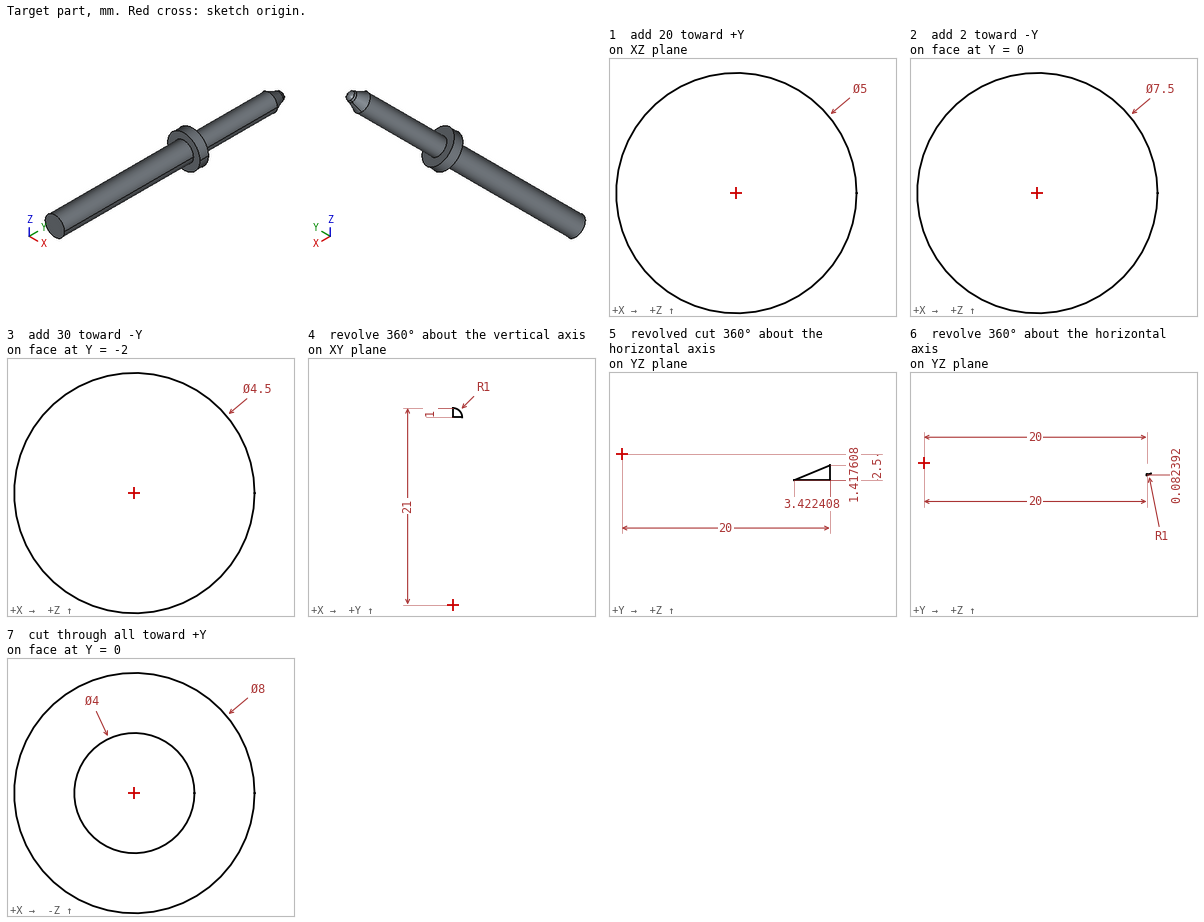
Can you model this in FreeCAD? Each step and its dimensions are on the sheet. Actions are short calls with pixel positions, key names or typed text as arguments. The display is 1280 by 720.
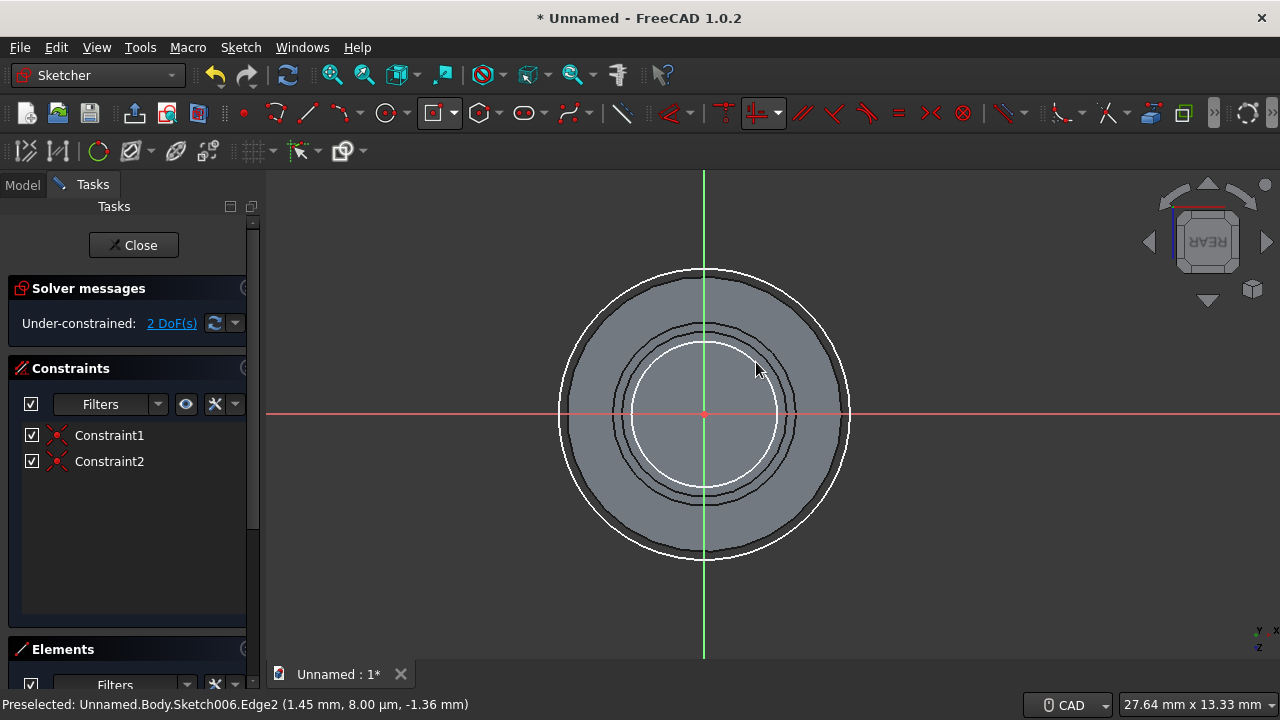
click(670, 114)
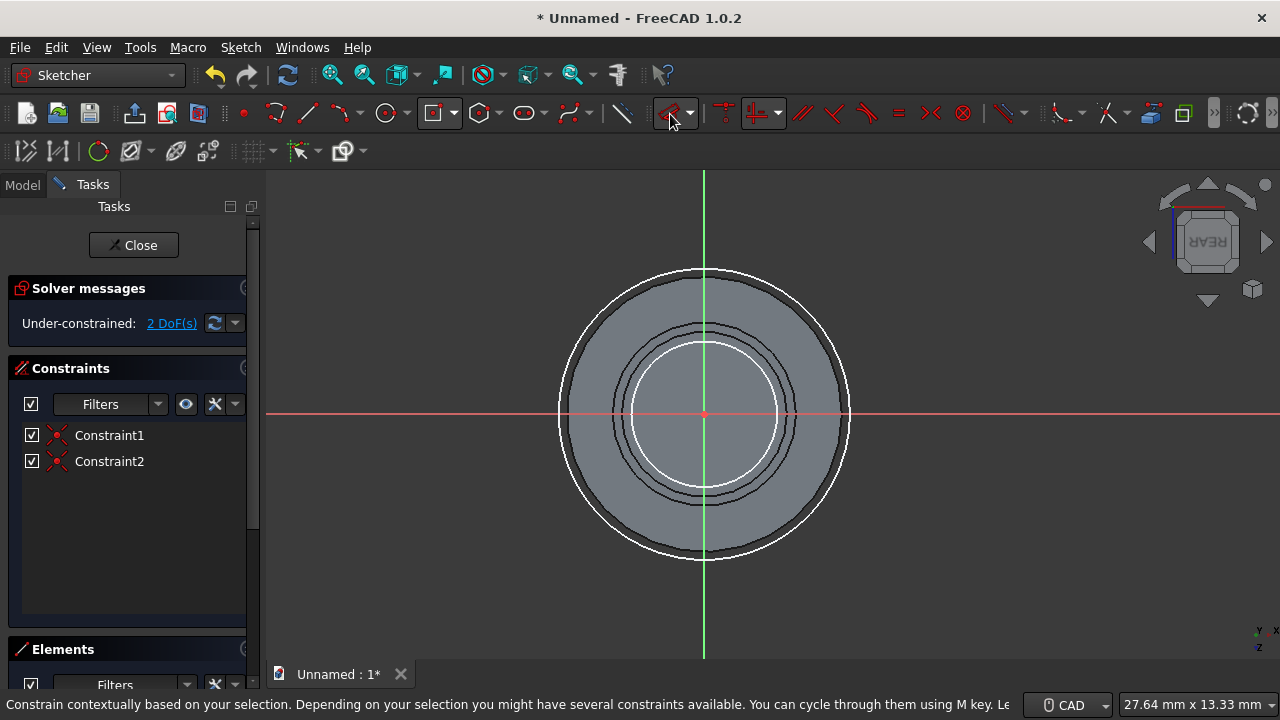
click(807, 311)
click(830, 288)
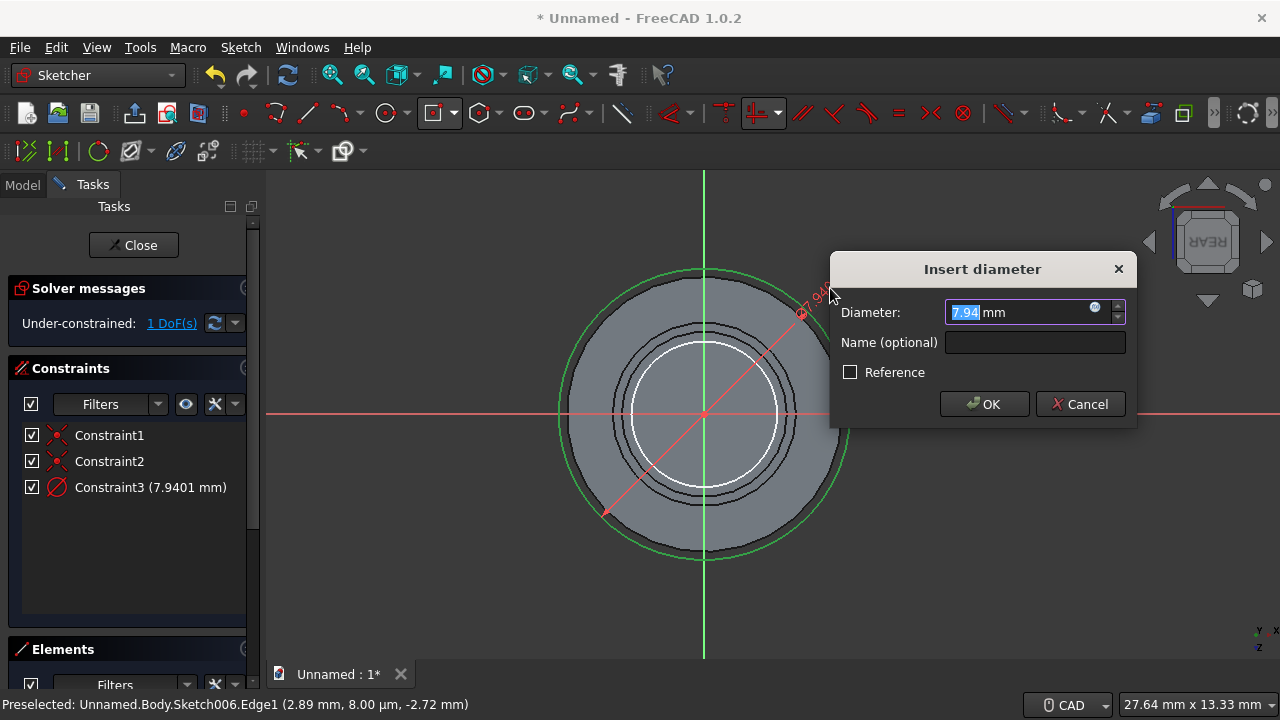
text(8)
key(Return)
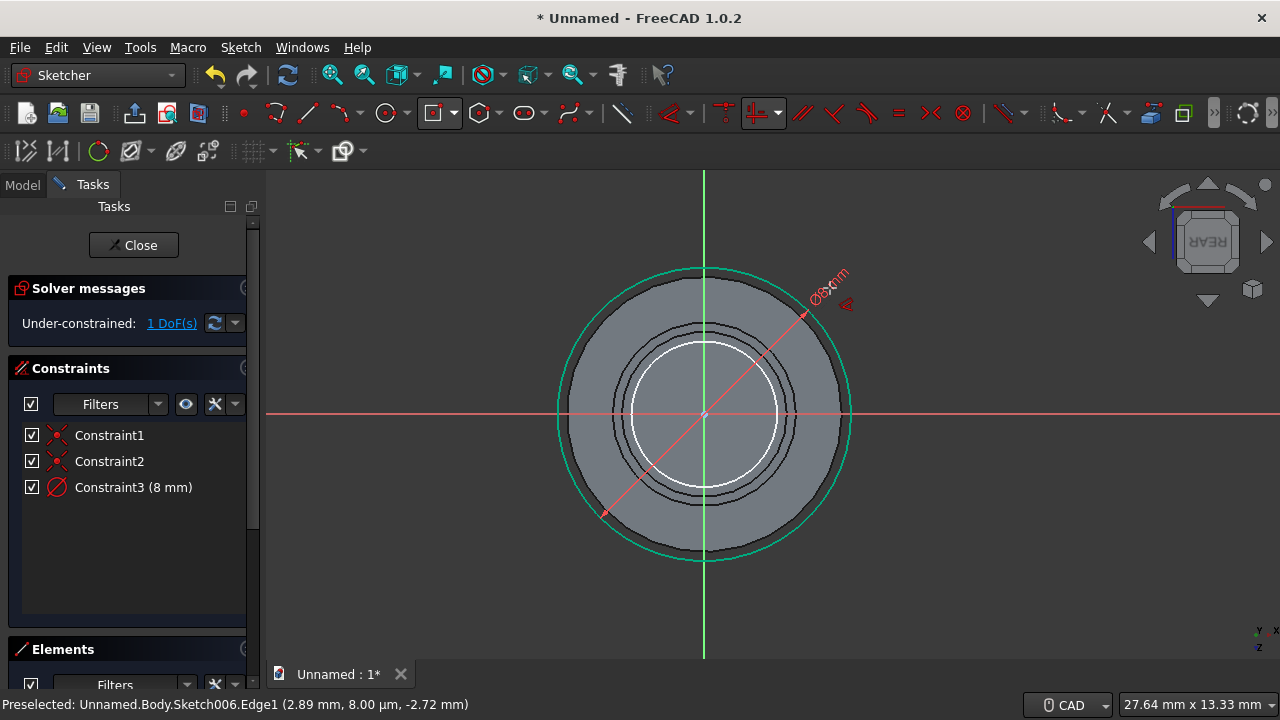
click(756, 363)
click(779, 340)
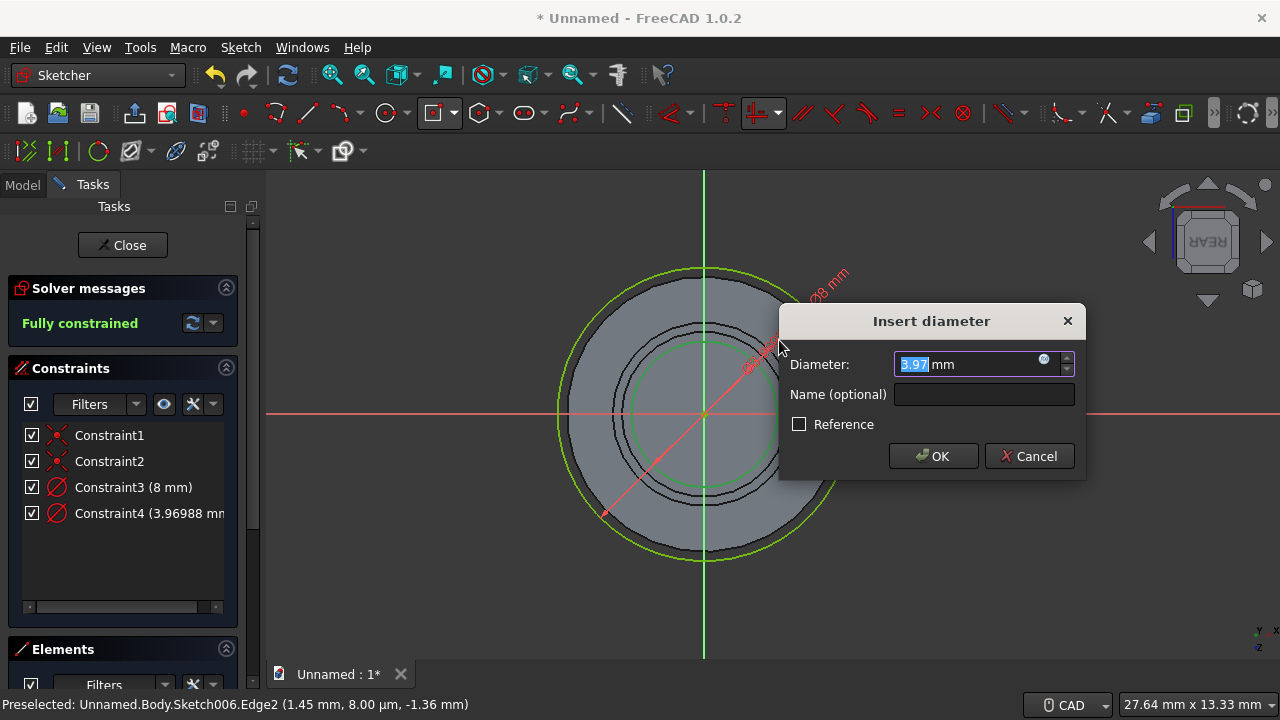
text(4)
key(Return)
key(Escape)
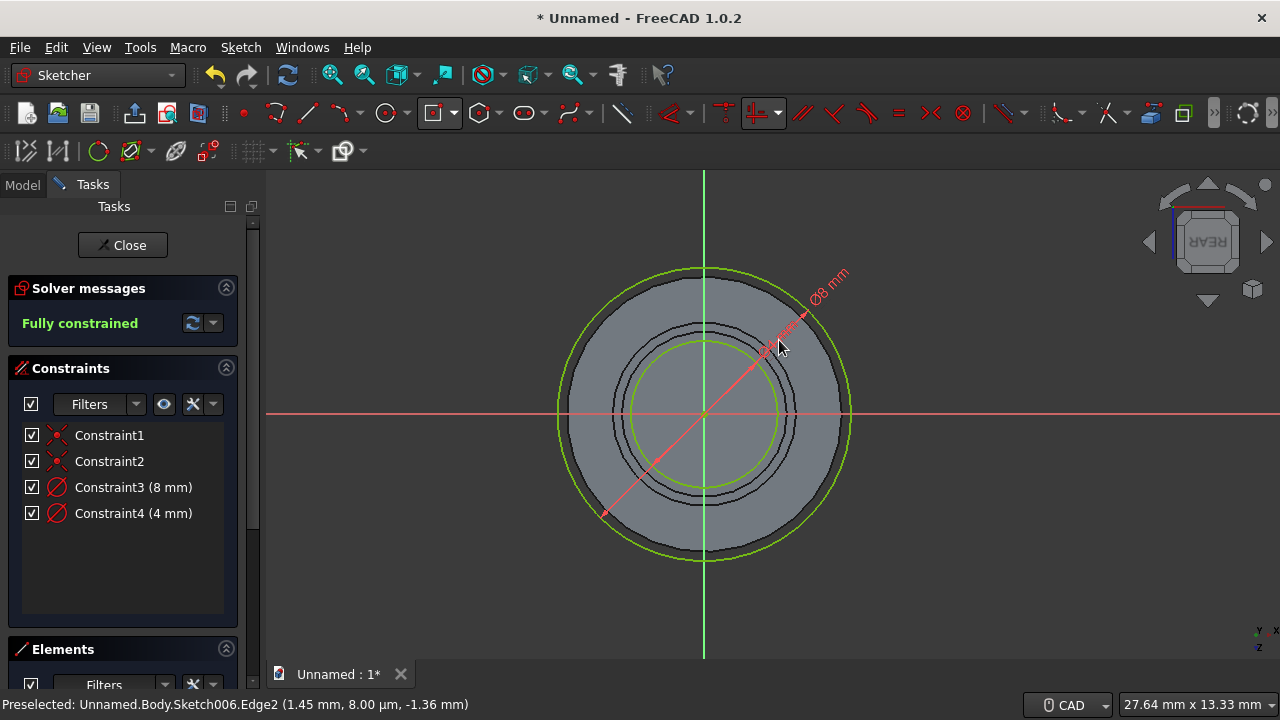
click(123, 245)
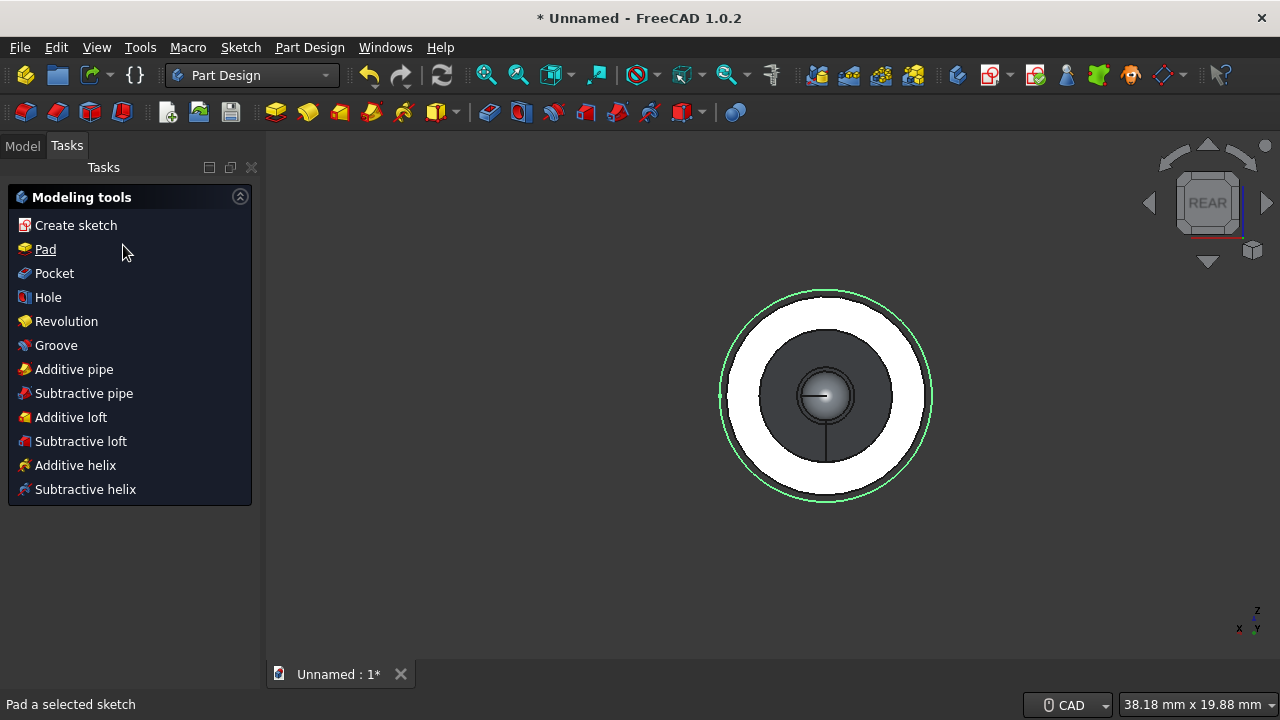
click(490, 112)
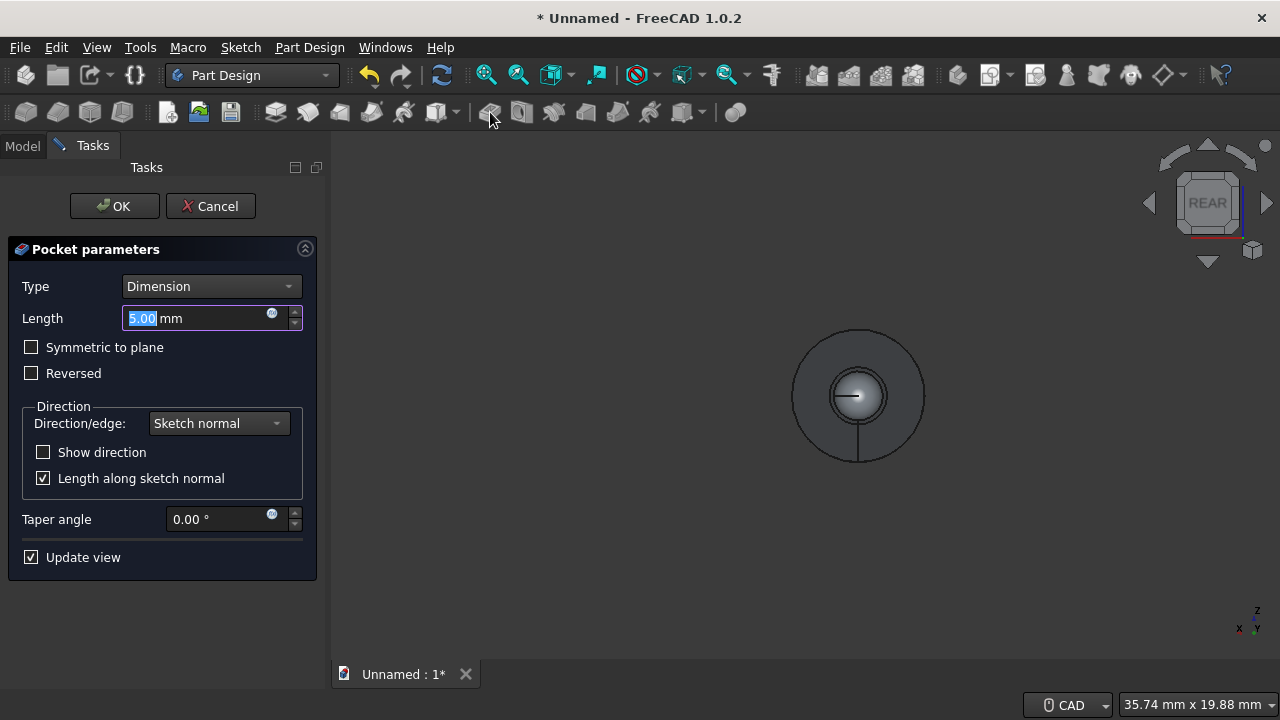
click(212, 286)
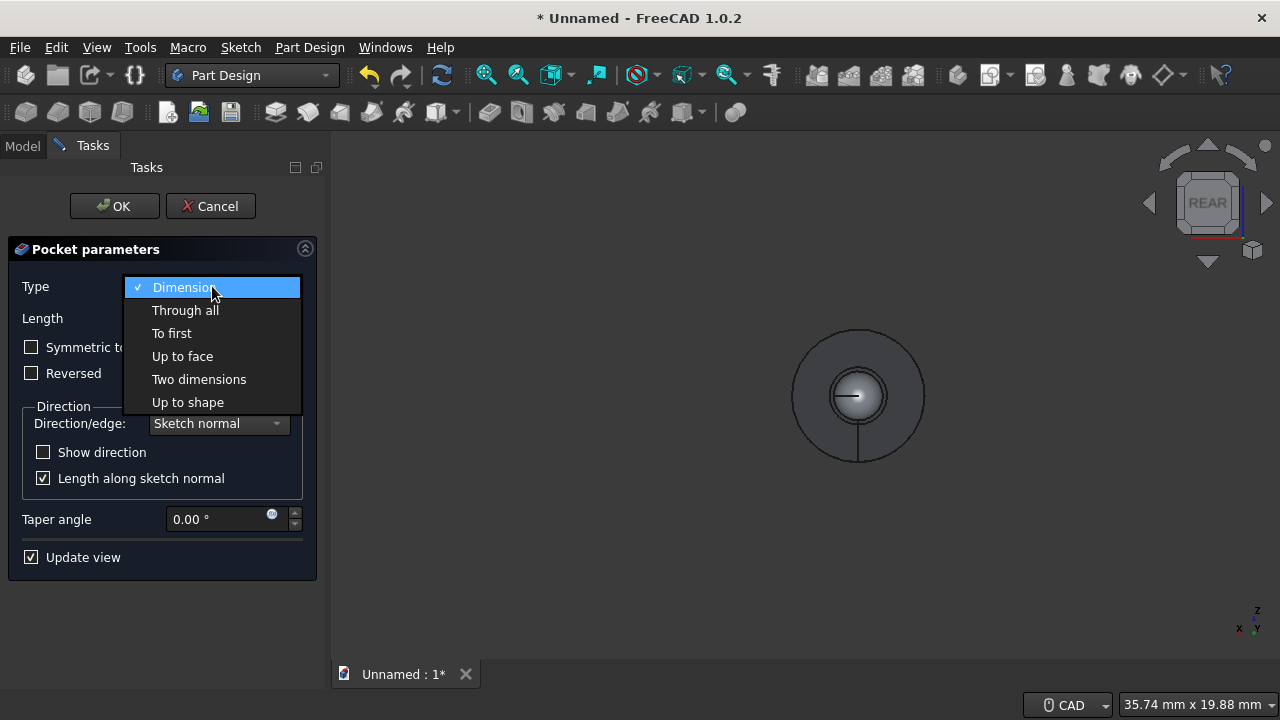
click(212, 310)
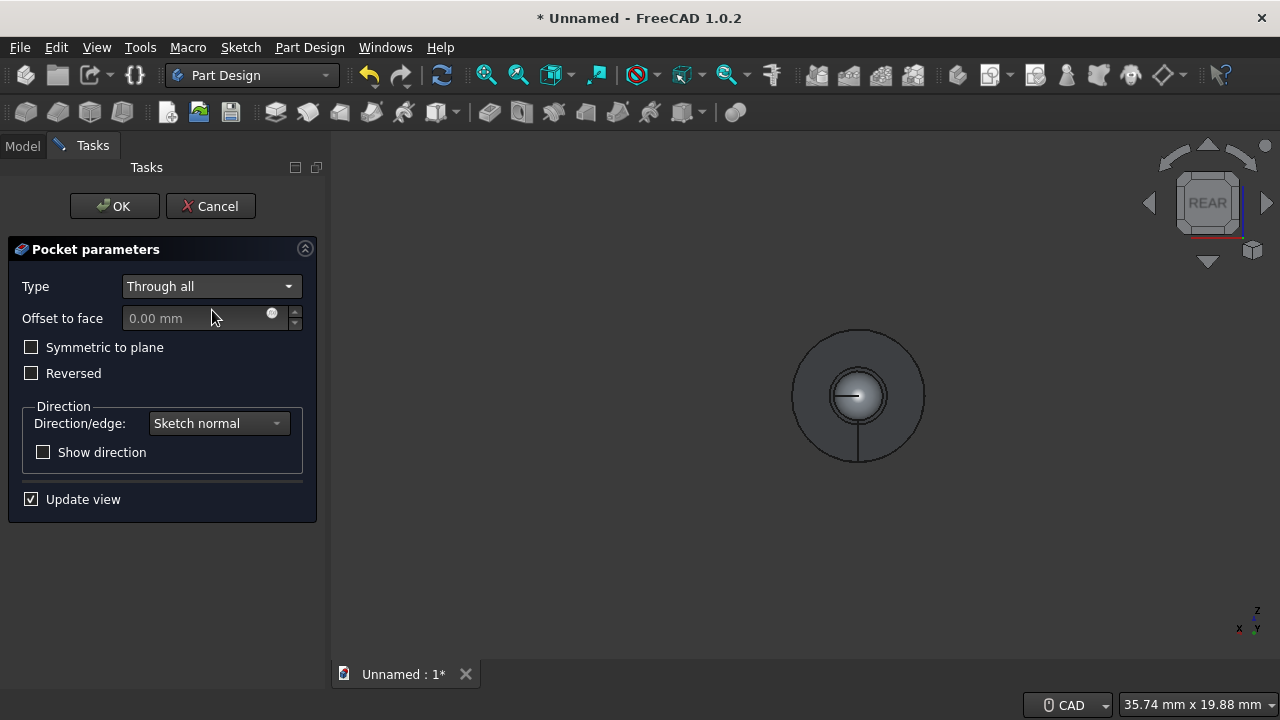
click(30, 373)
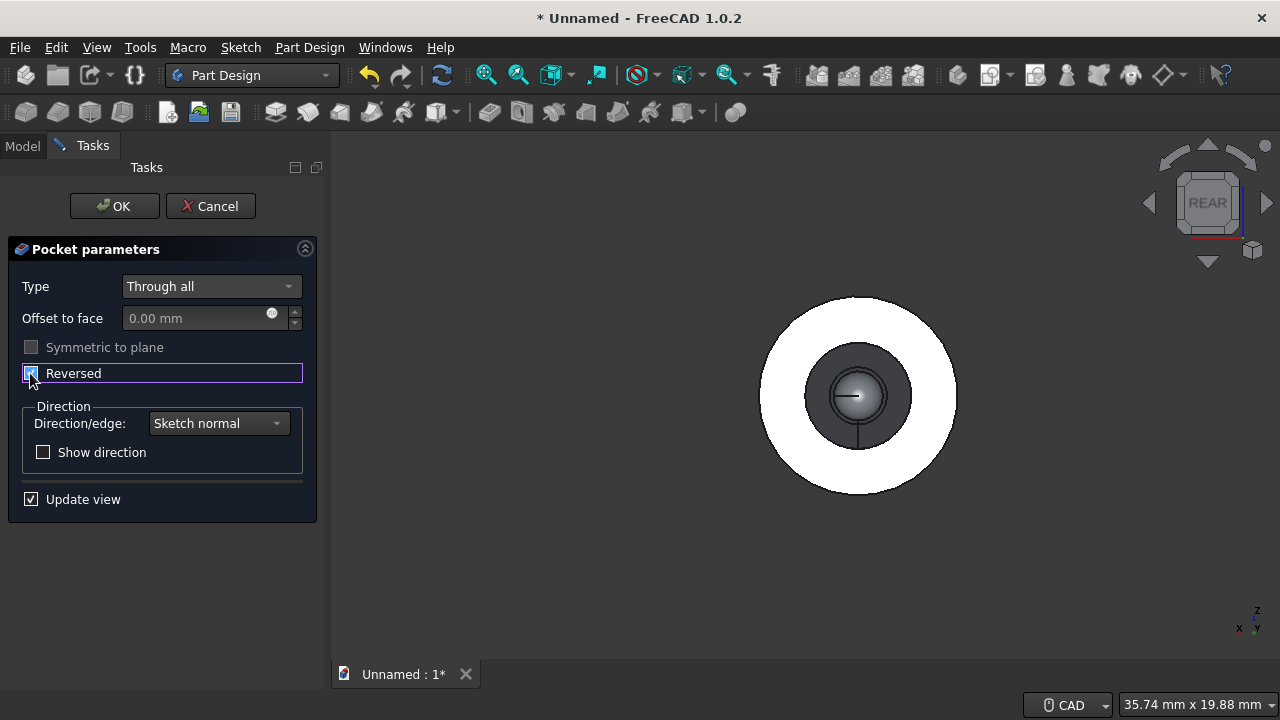
click(115, 206)